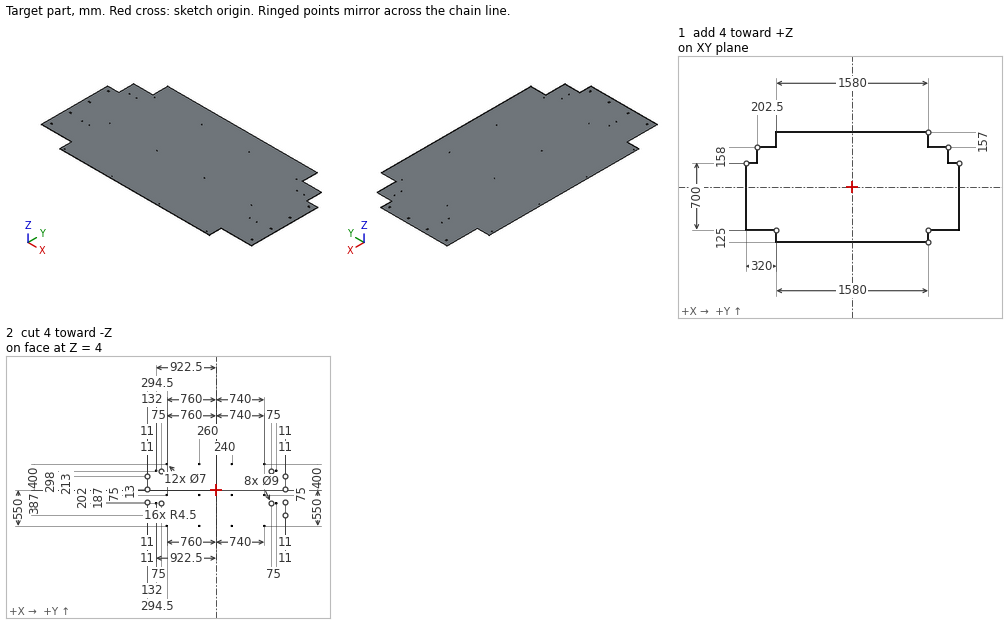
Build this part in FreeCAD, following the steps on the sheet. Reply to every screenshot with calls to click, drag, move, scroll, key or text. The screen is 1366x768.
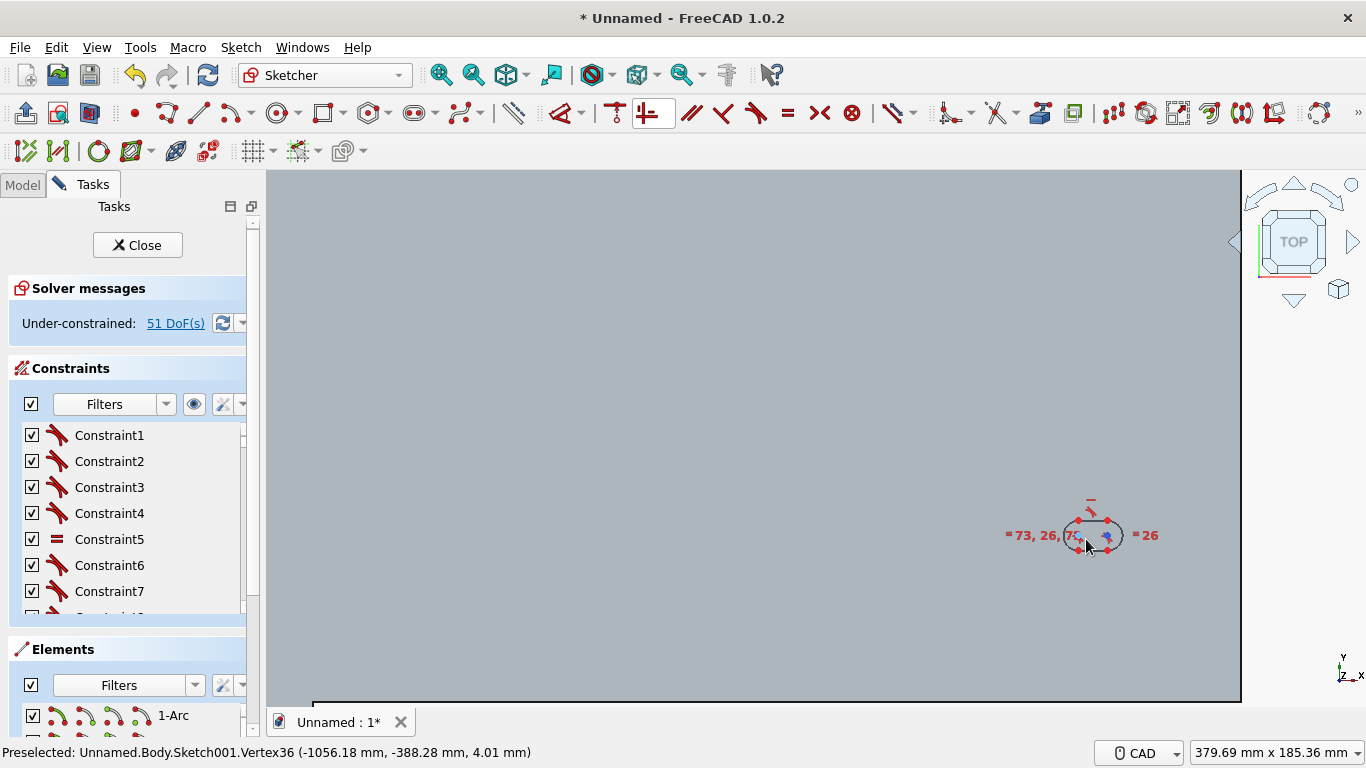
click(1078, 536)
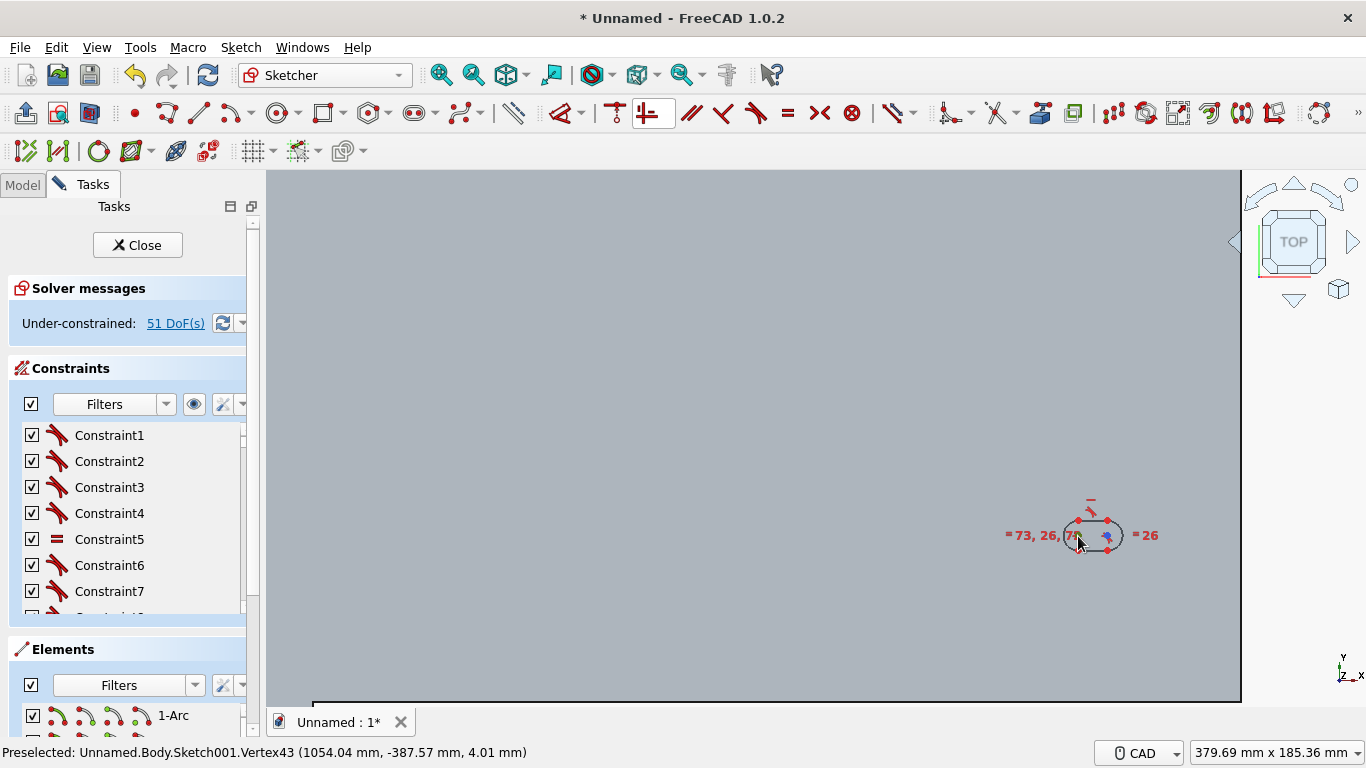
scroll(1087, 539, down, 11)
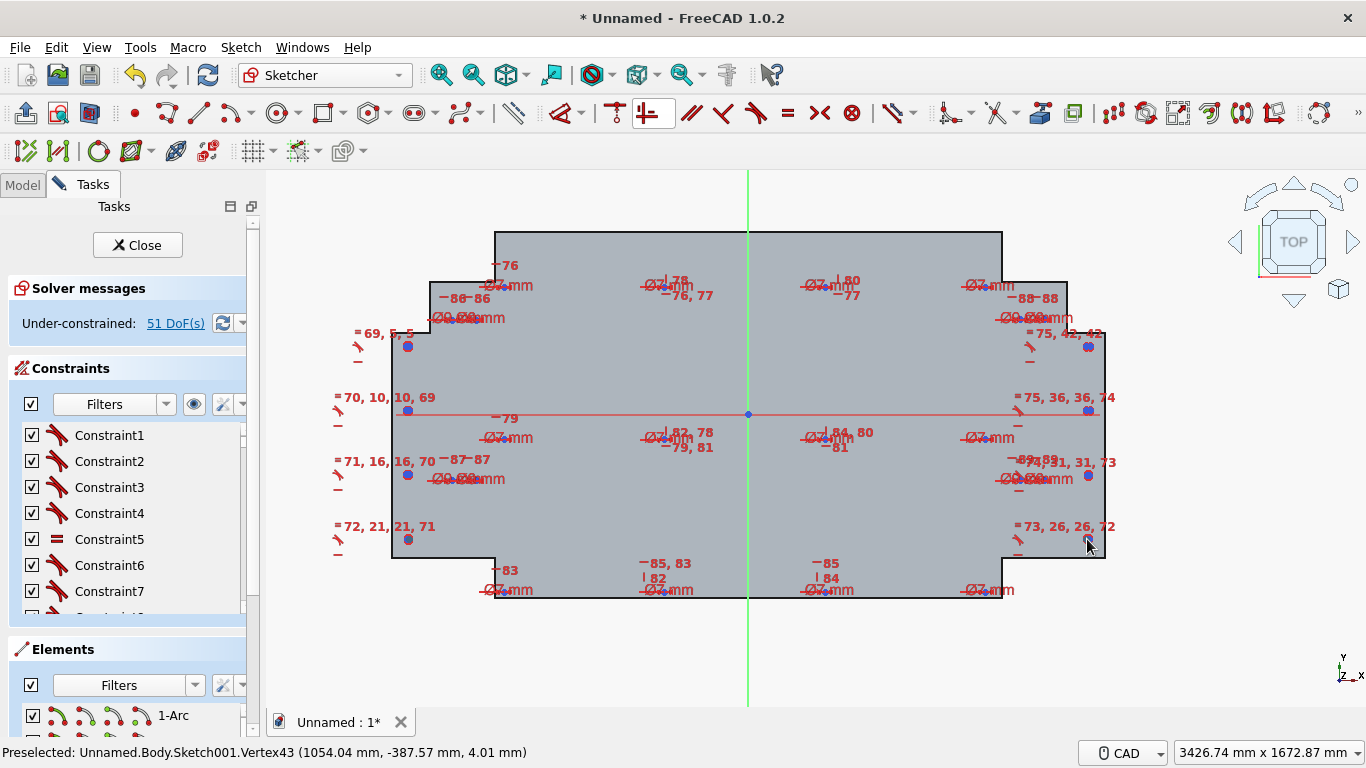
click(748, 645)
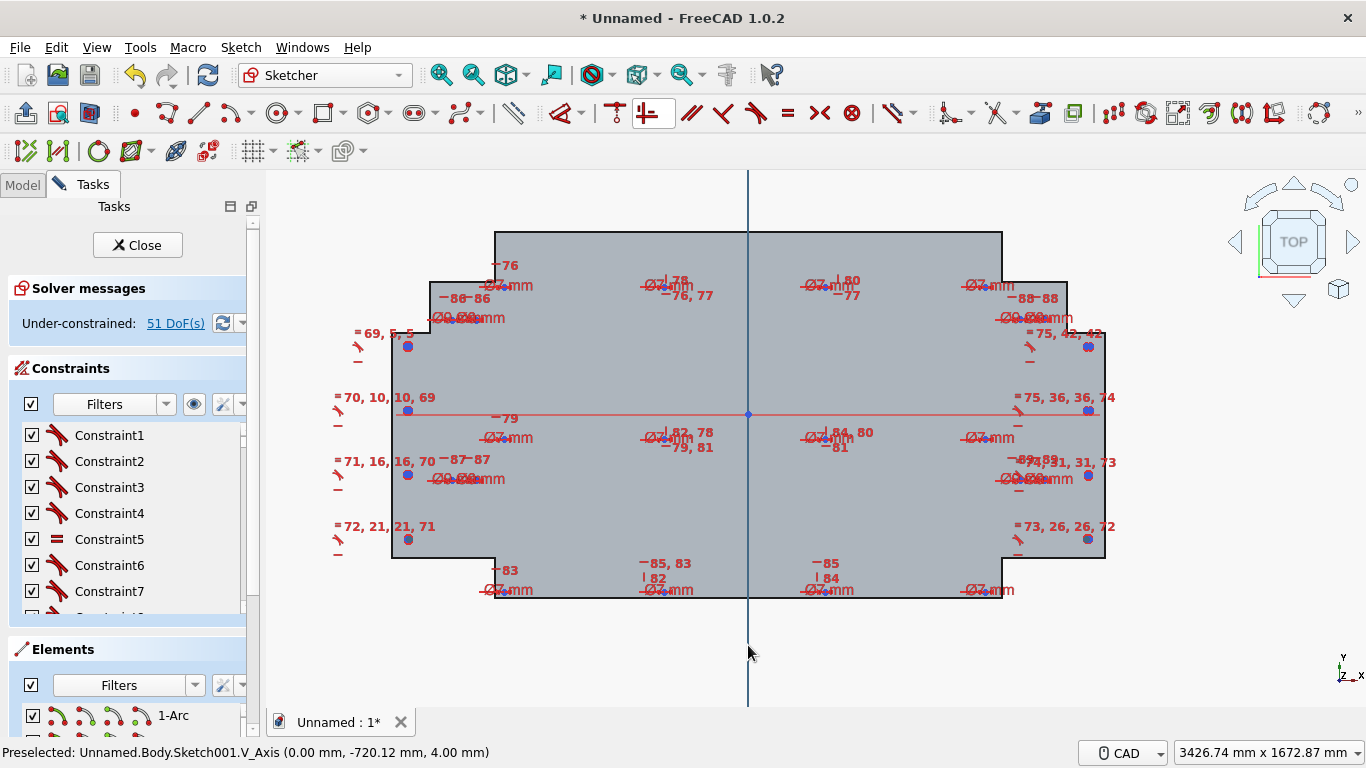
click(820, 114)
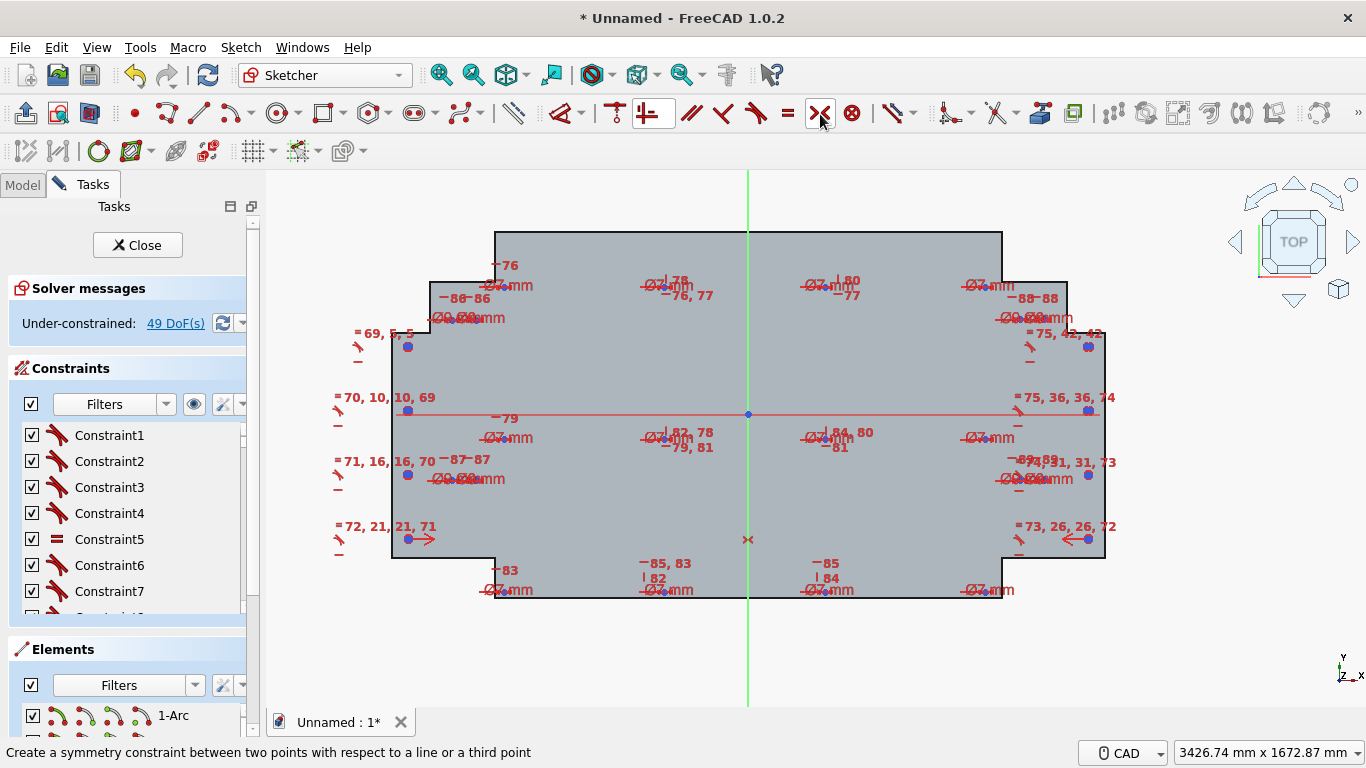
scroll(410, 475, up, 11)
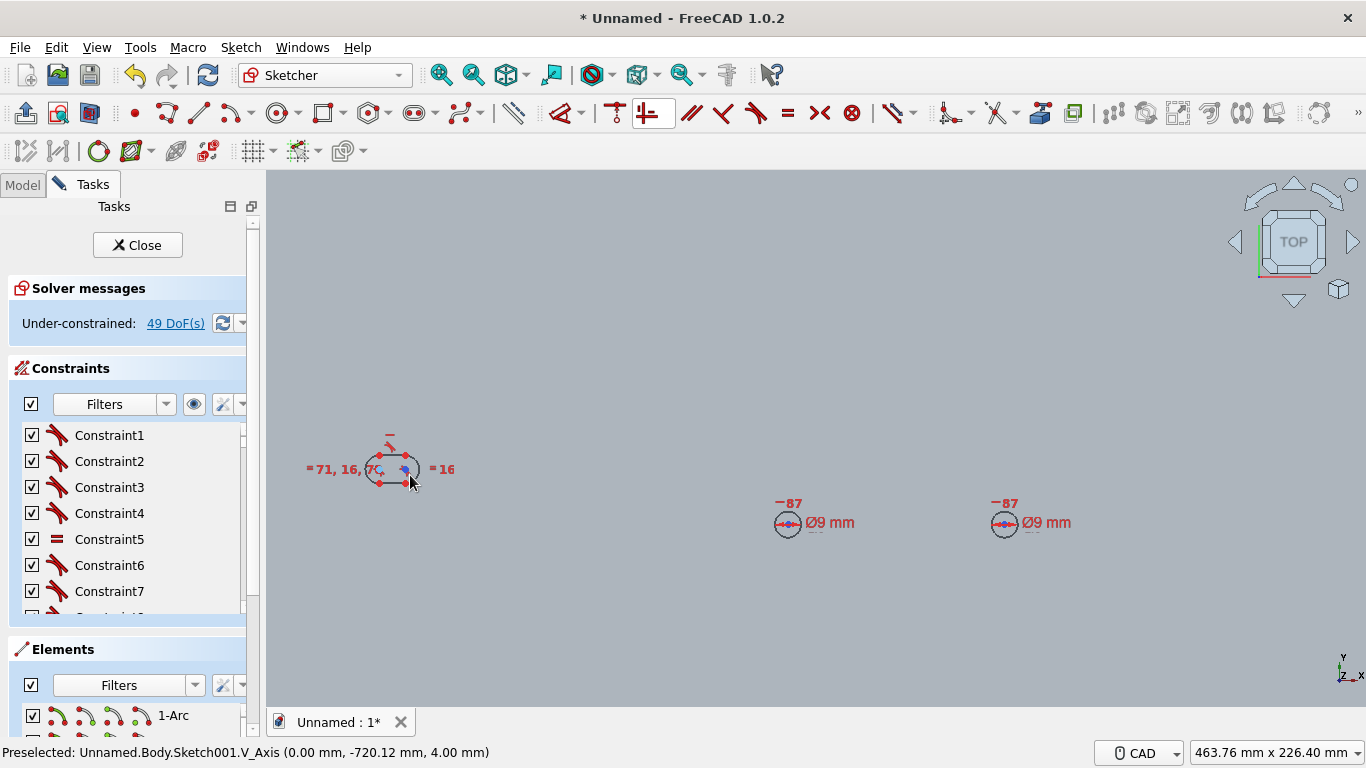
click(405, 469)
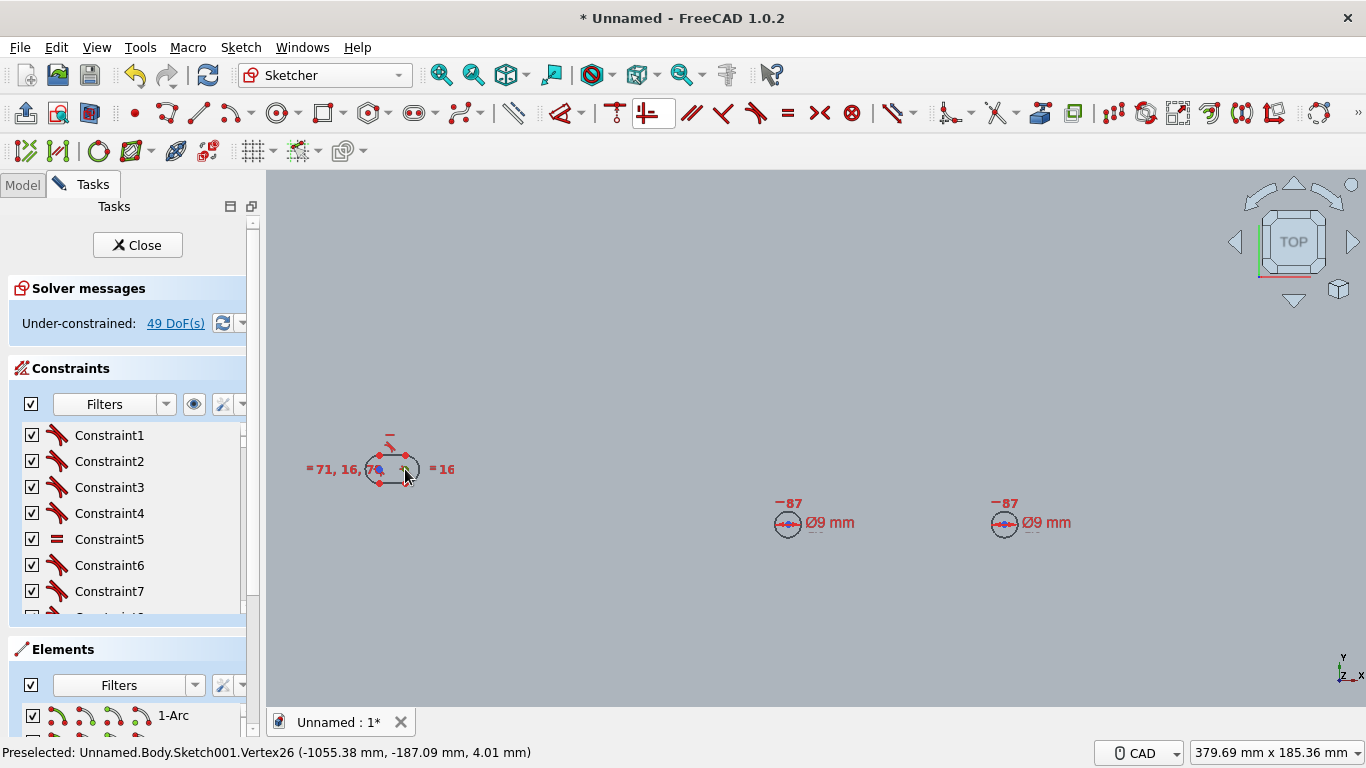
scroll(409, 475, down, 11)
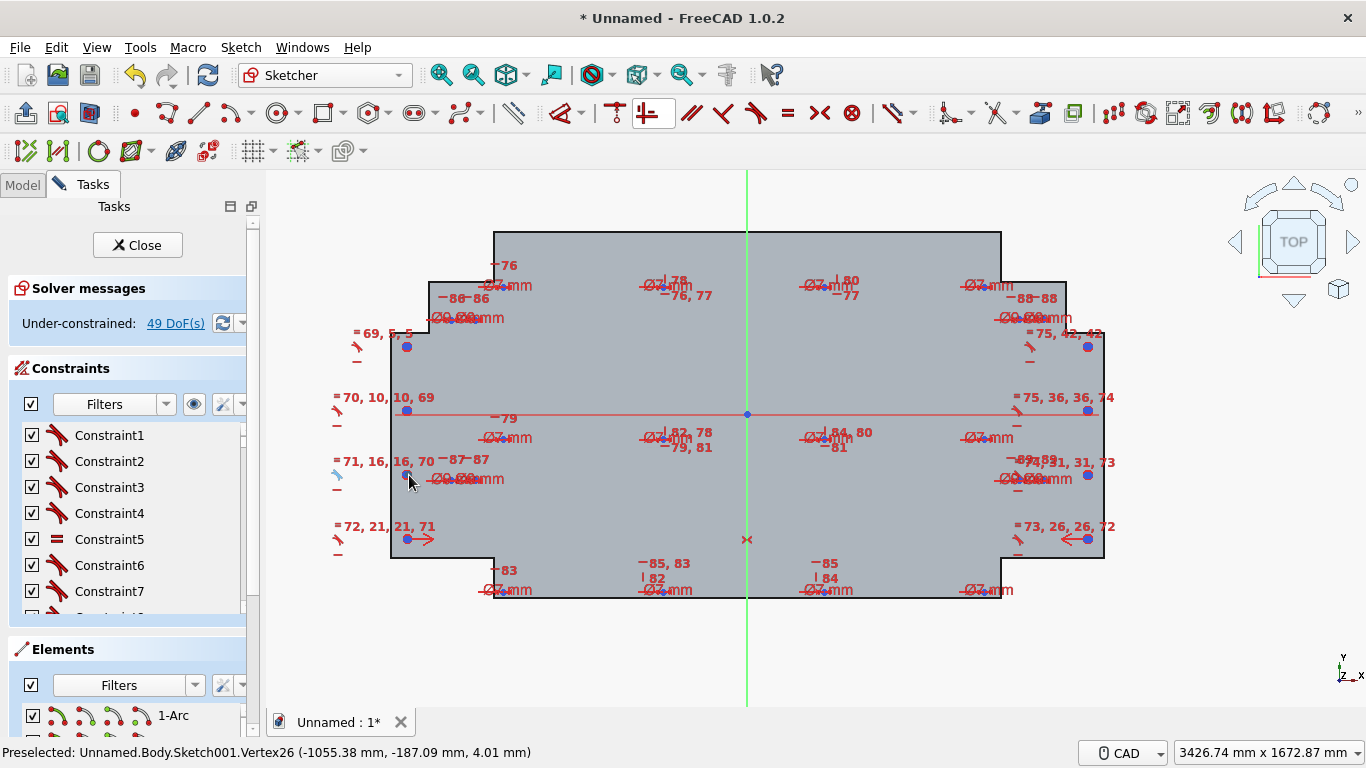
scroll(1087, 475, up, 11)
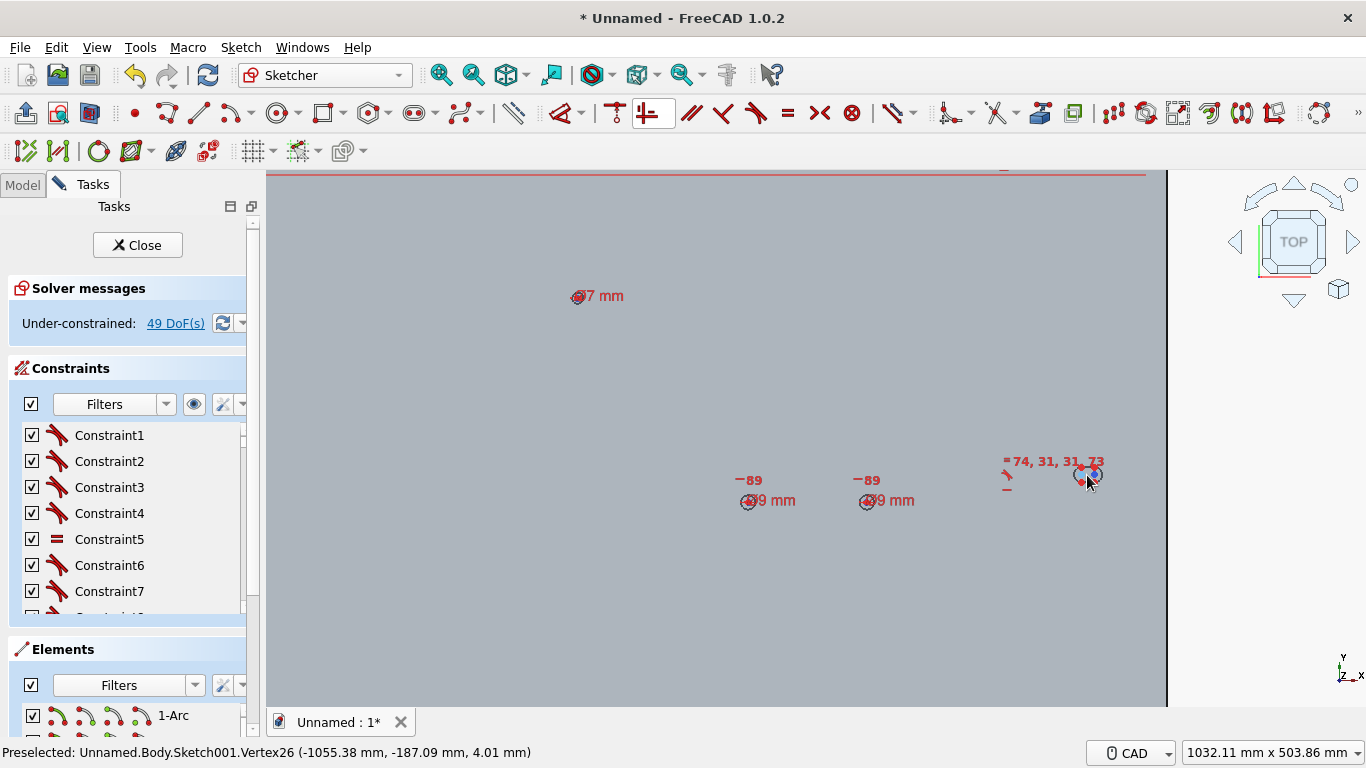
click(1077, 474)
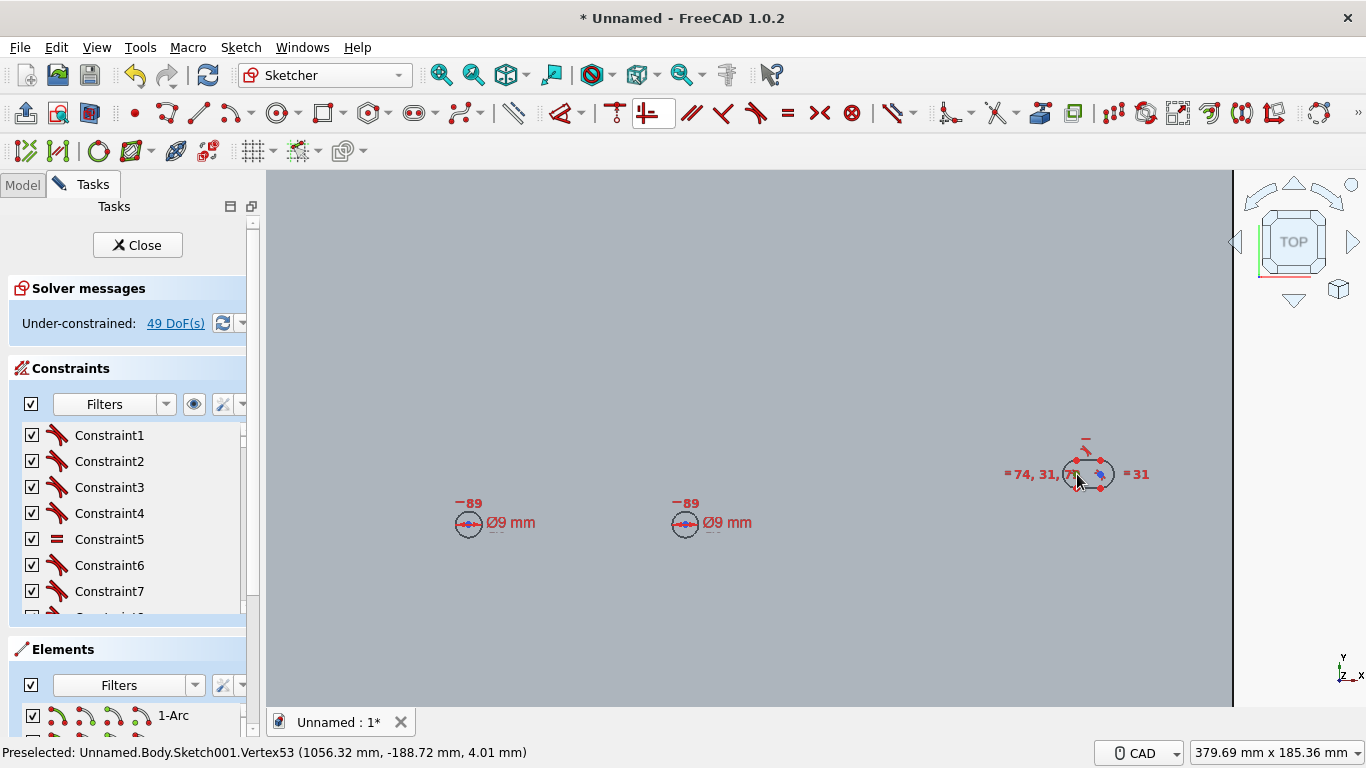
scroll(1088, 475, down, 11)